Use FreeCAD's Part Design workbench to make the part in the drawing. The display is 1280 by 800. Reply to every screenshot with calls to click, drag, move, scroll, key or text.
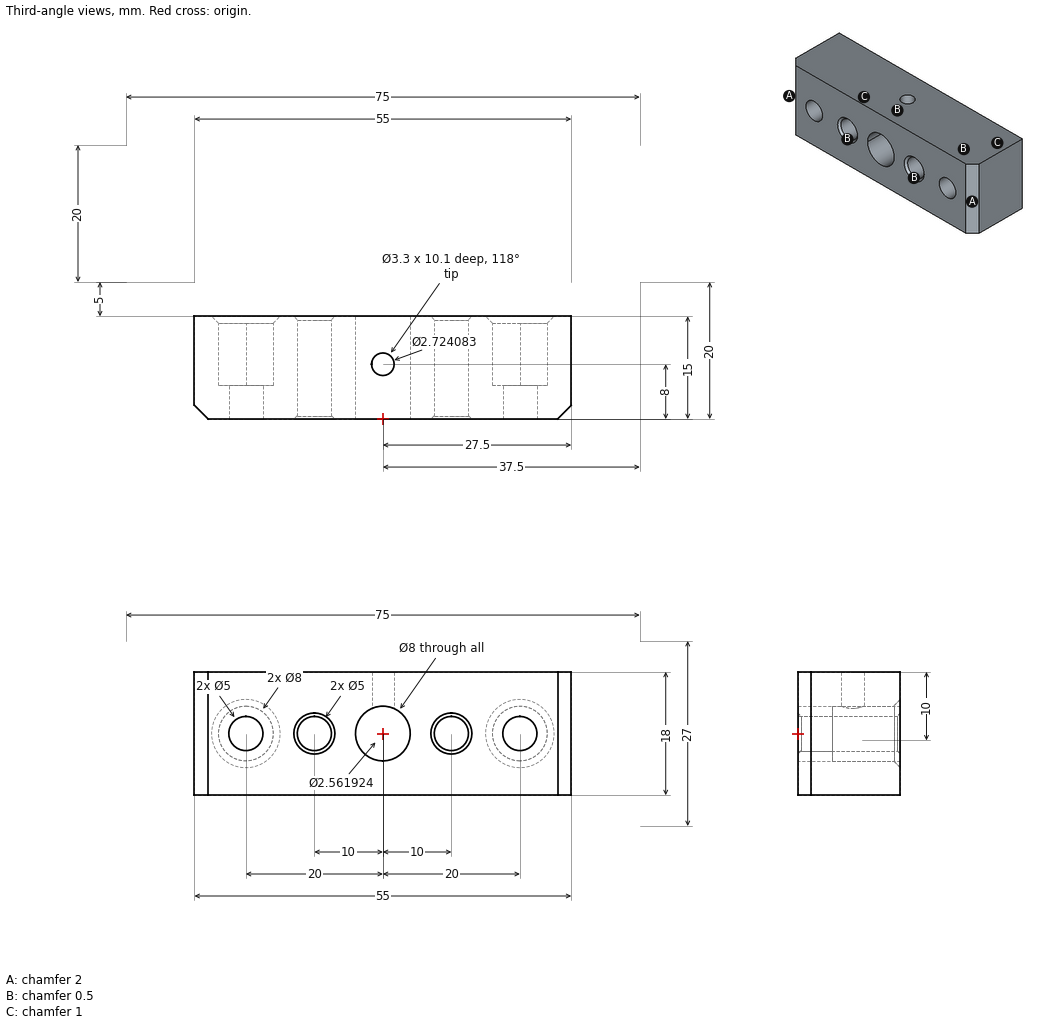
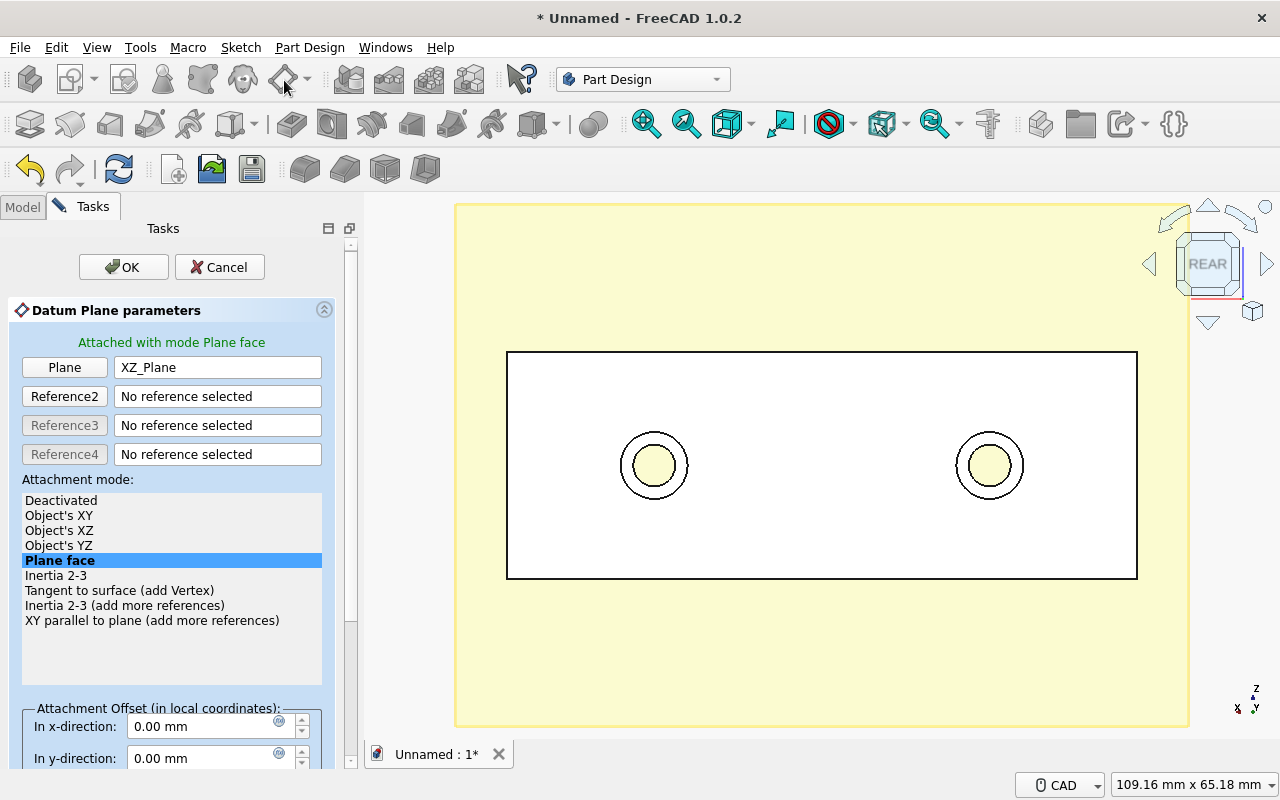
scroll(351, 503, down, 2)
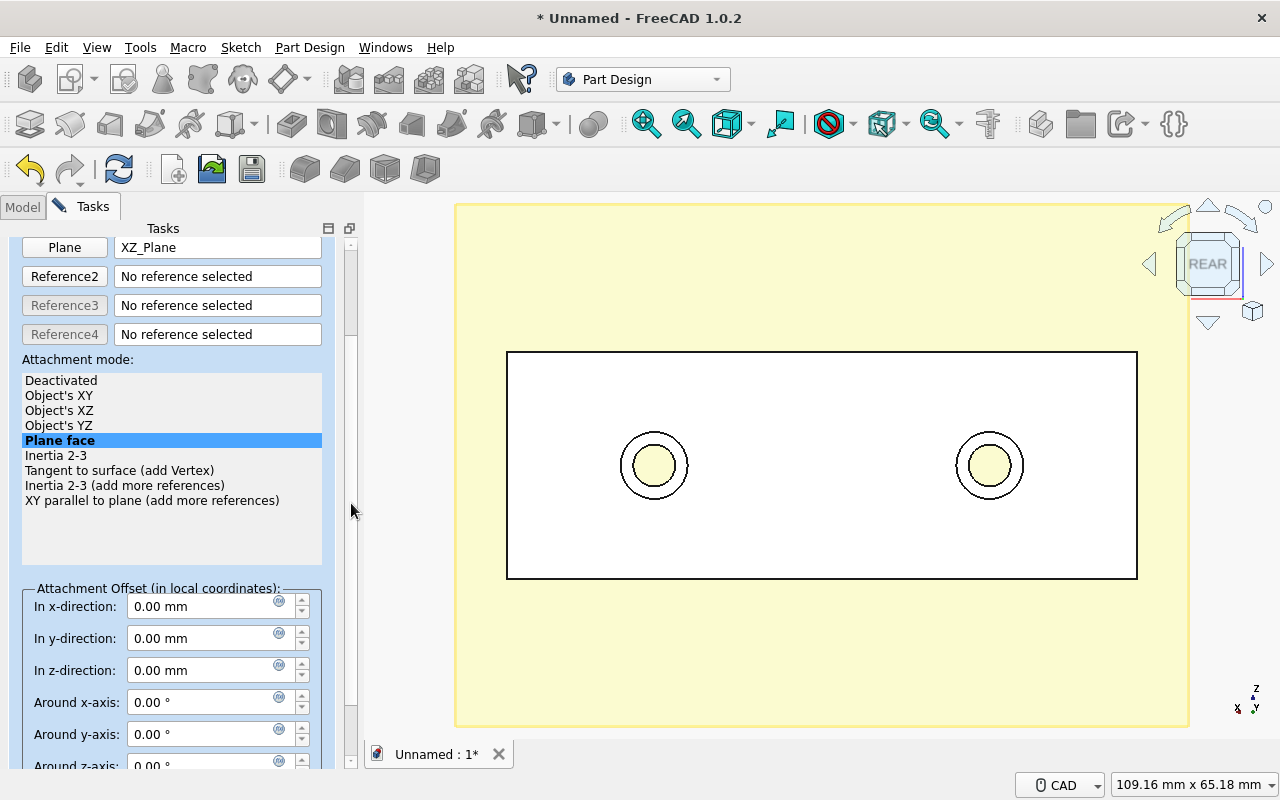
triple_click(210, 670)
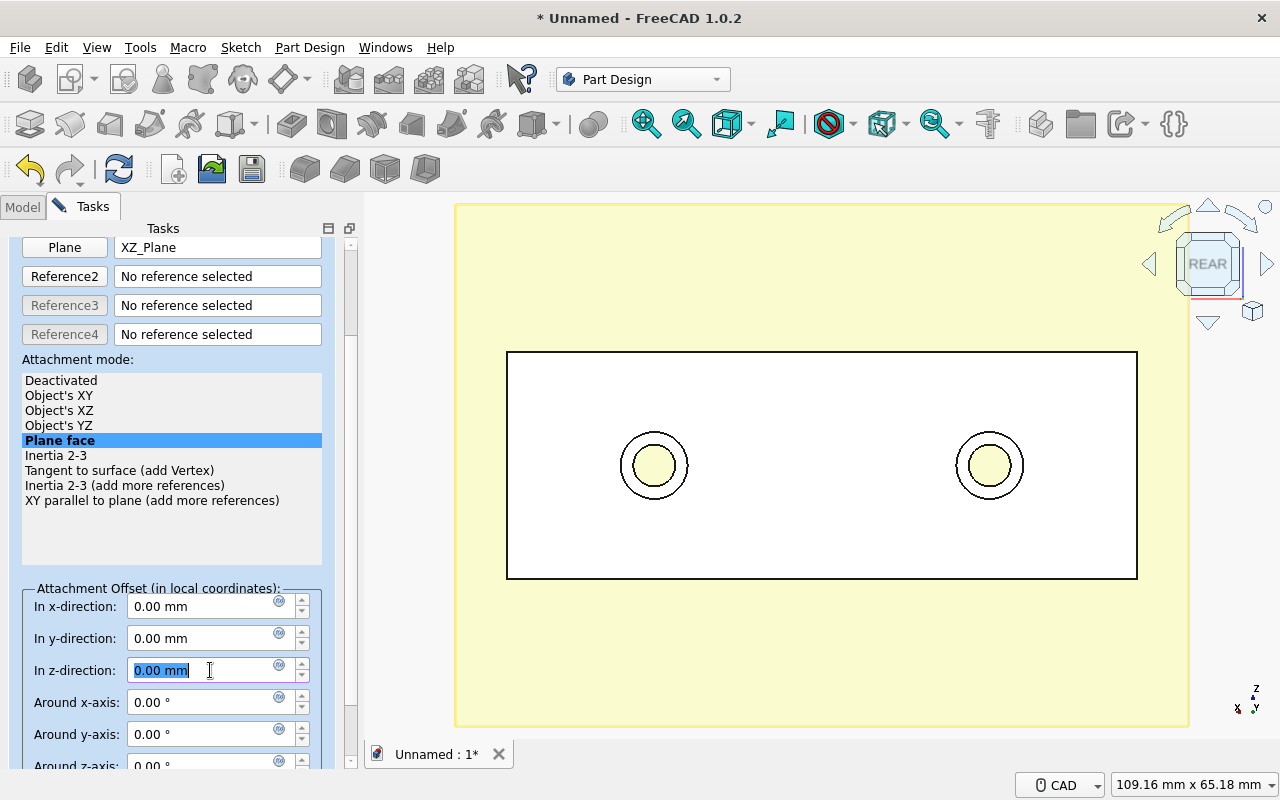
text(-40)
key(Tab)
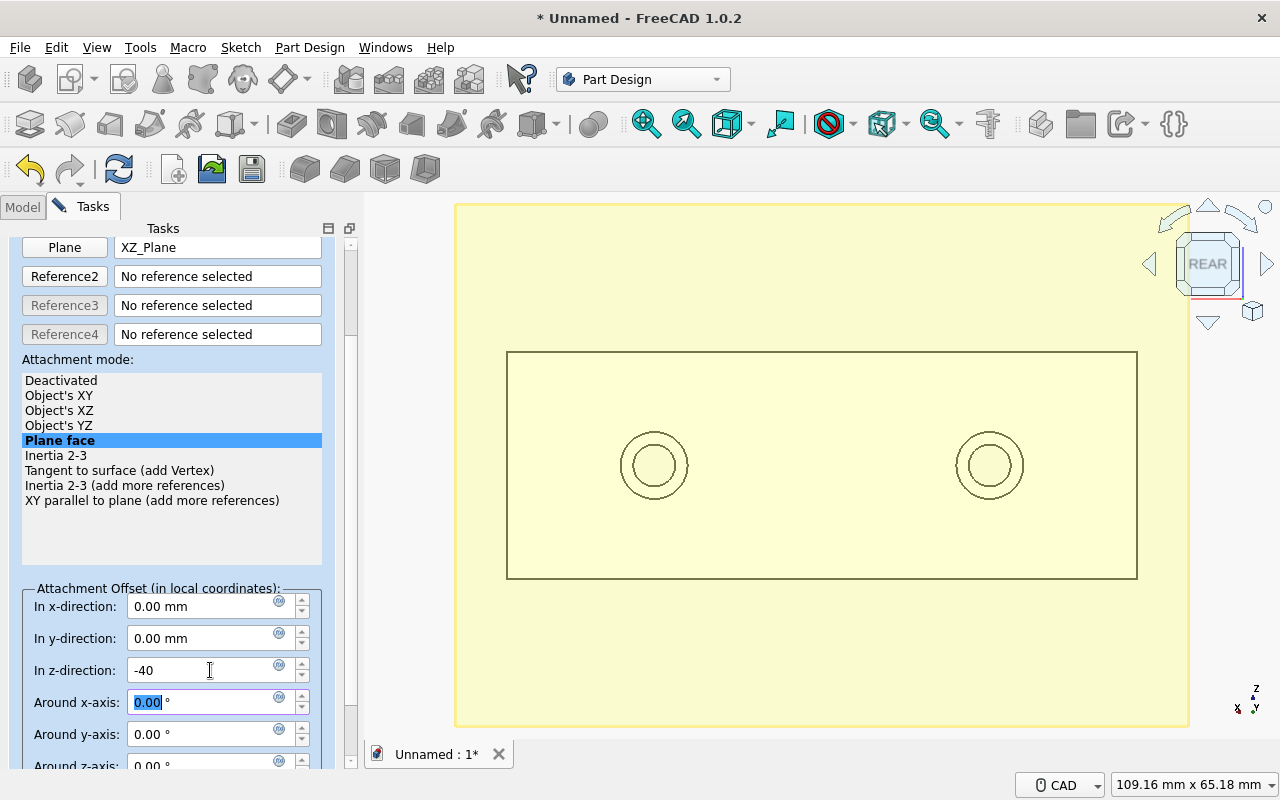
scroll(351, 503, up, 3)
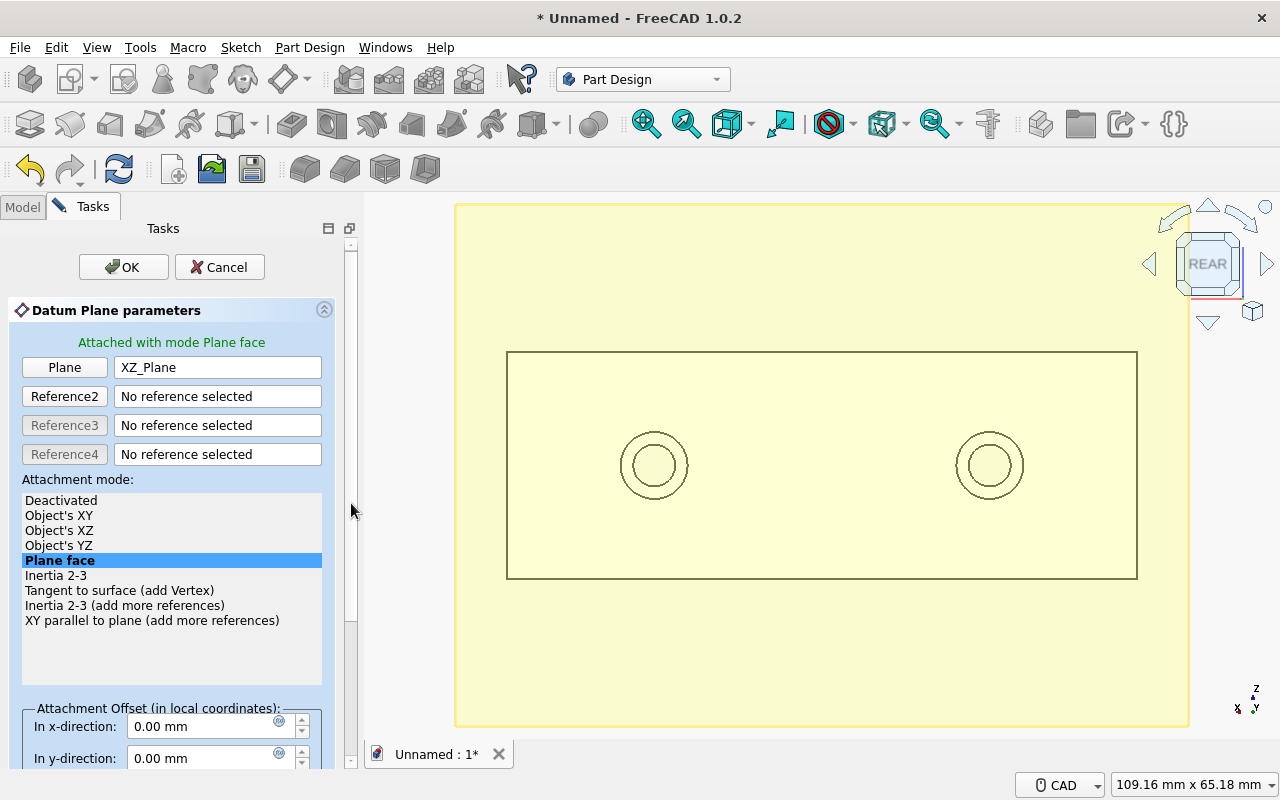
click(124, 267)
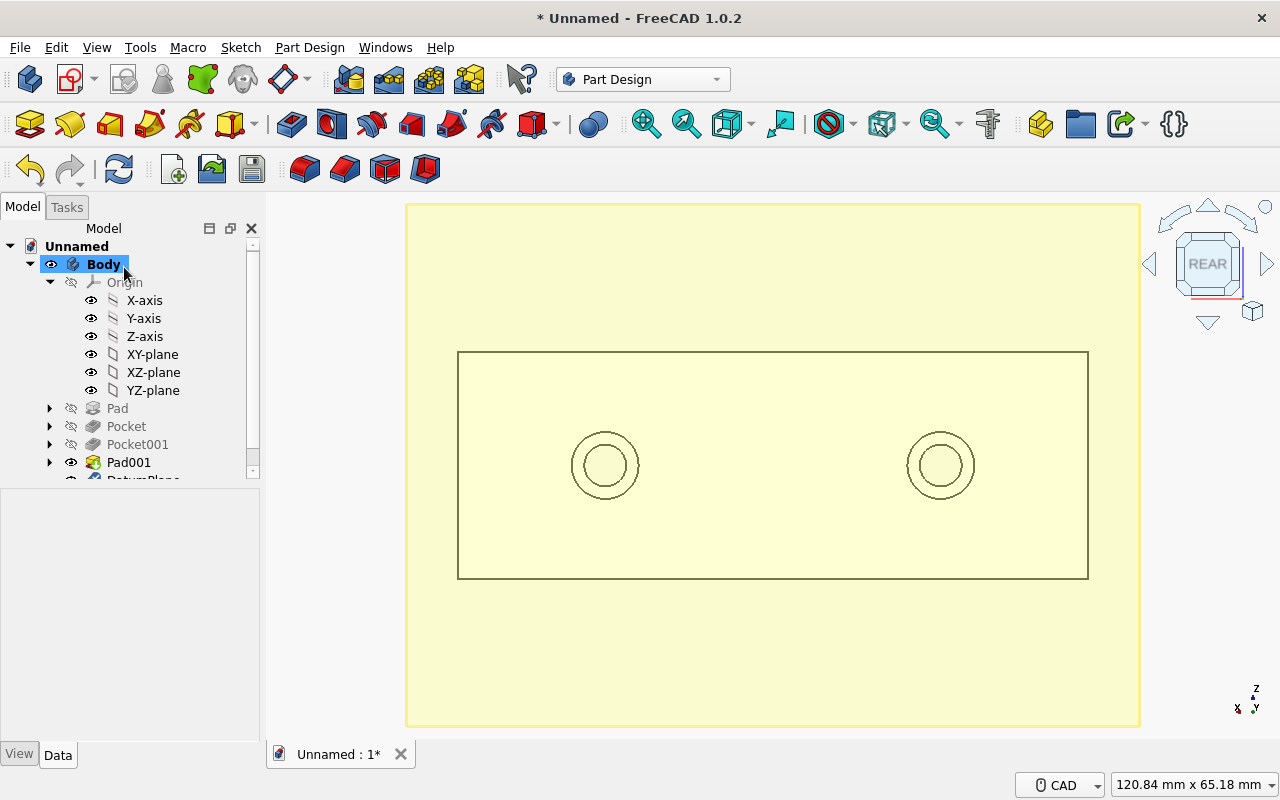
scroll(100, 350, down, 3)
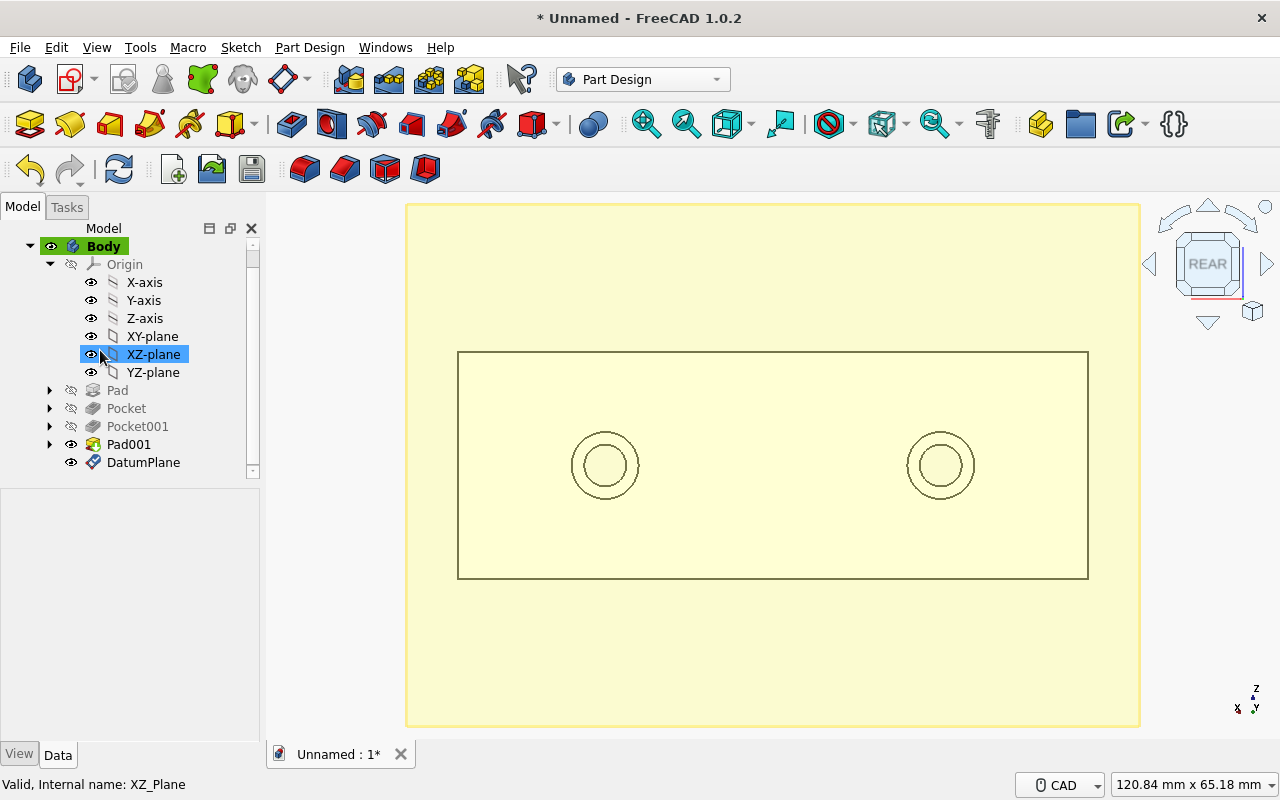
click(116, 462)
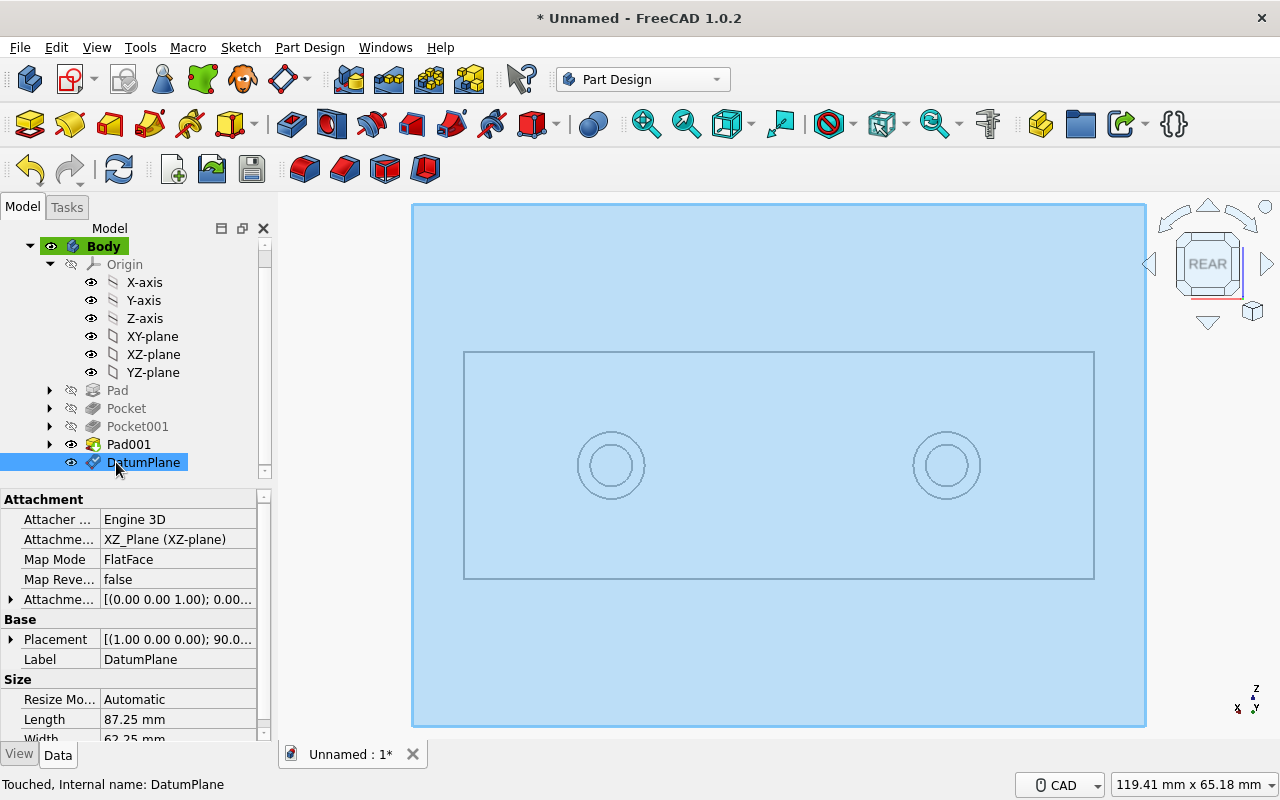
click(70, 80)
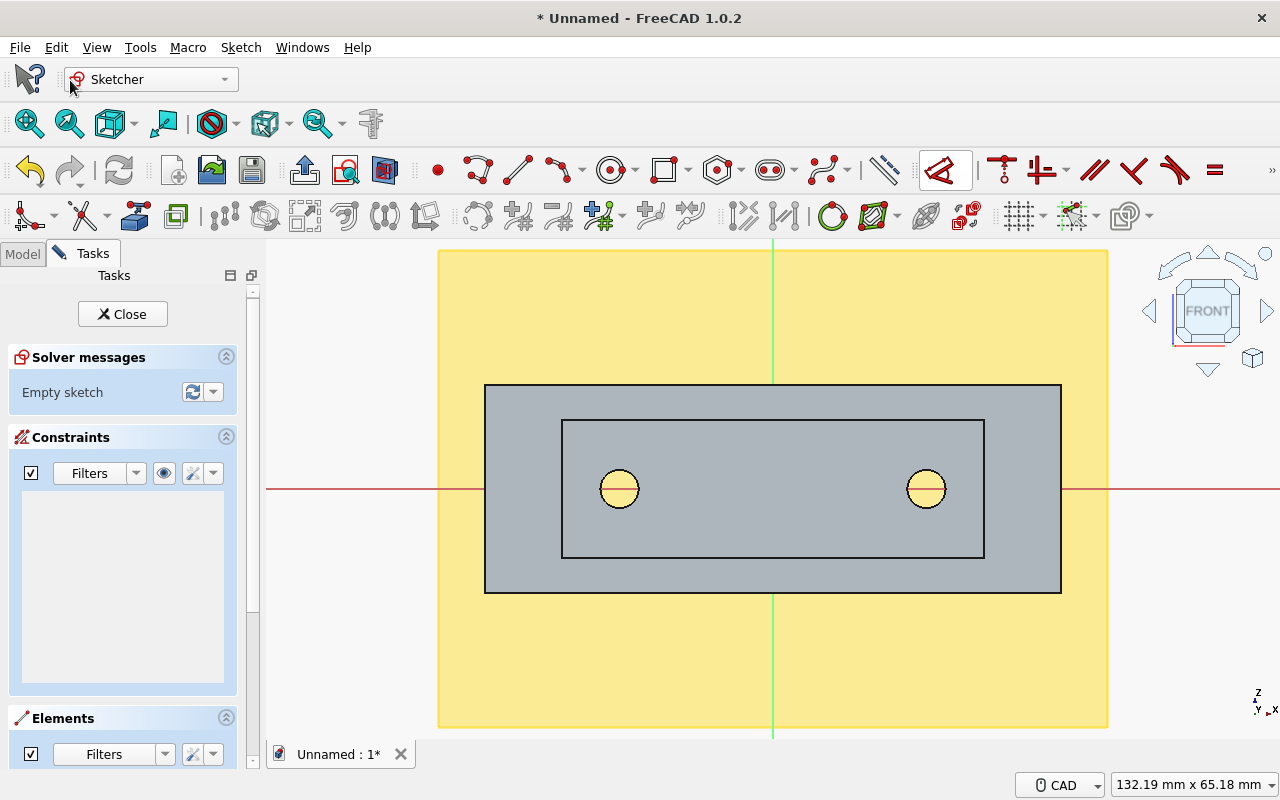
click(386, 170)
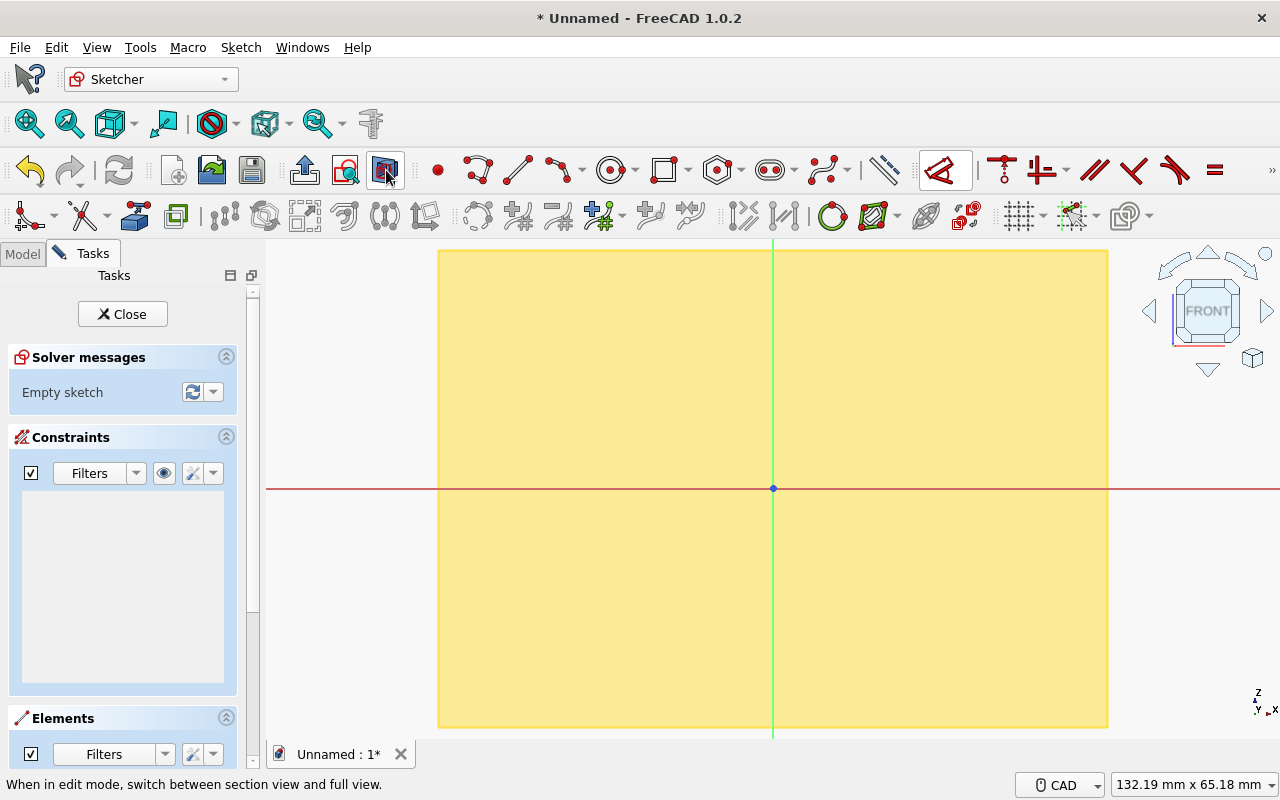
key(g)
key(v)